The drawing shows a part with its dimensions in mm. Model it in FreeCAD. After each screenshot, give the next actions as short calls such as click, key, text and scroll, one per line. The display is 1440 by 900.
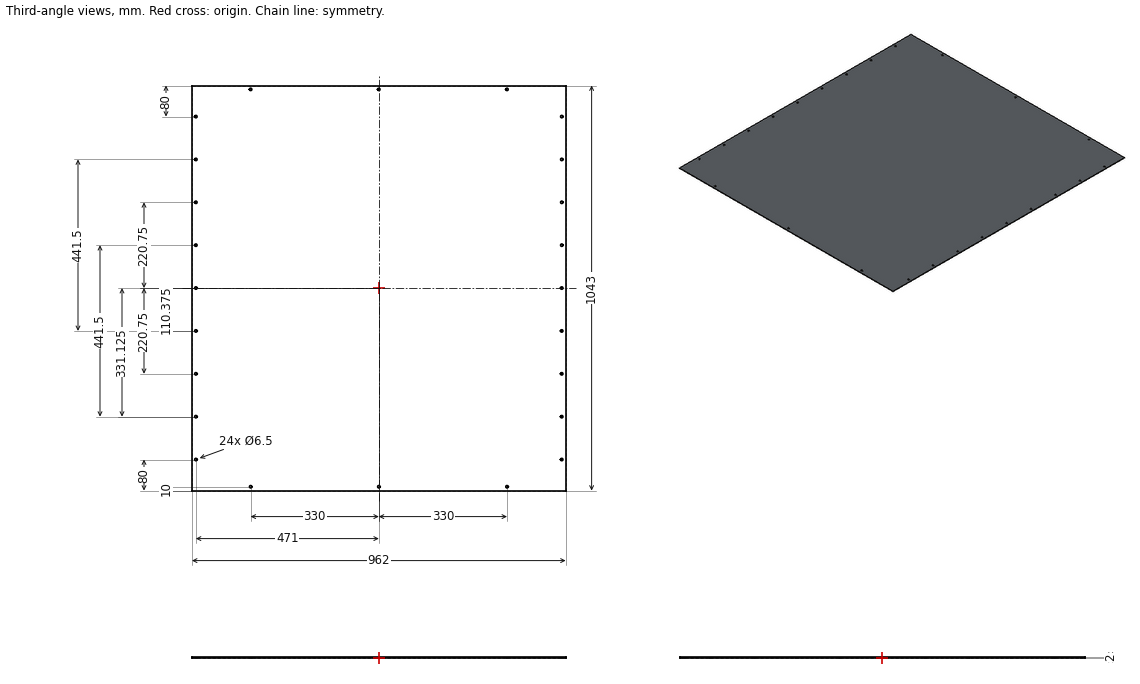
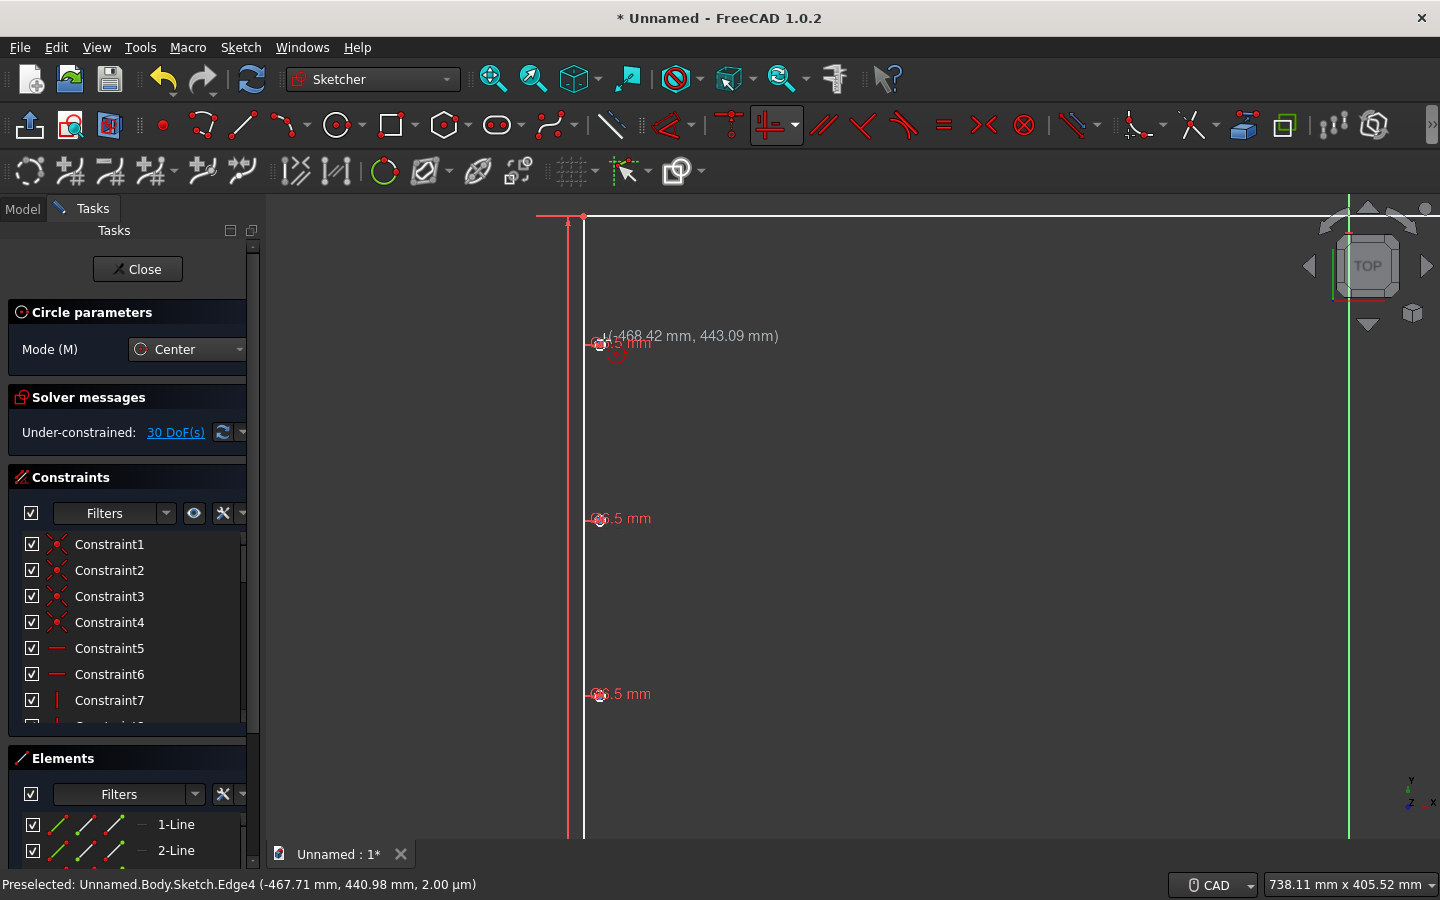
scroll(824, 232, up, 8)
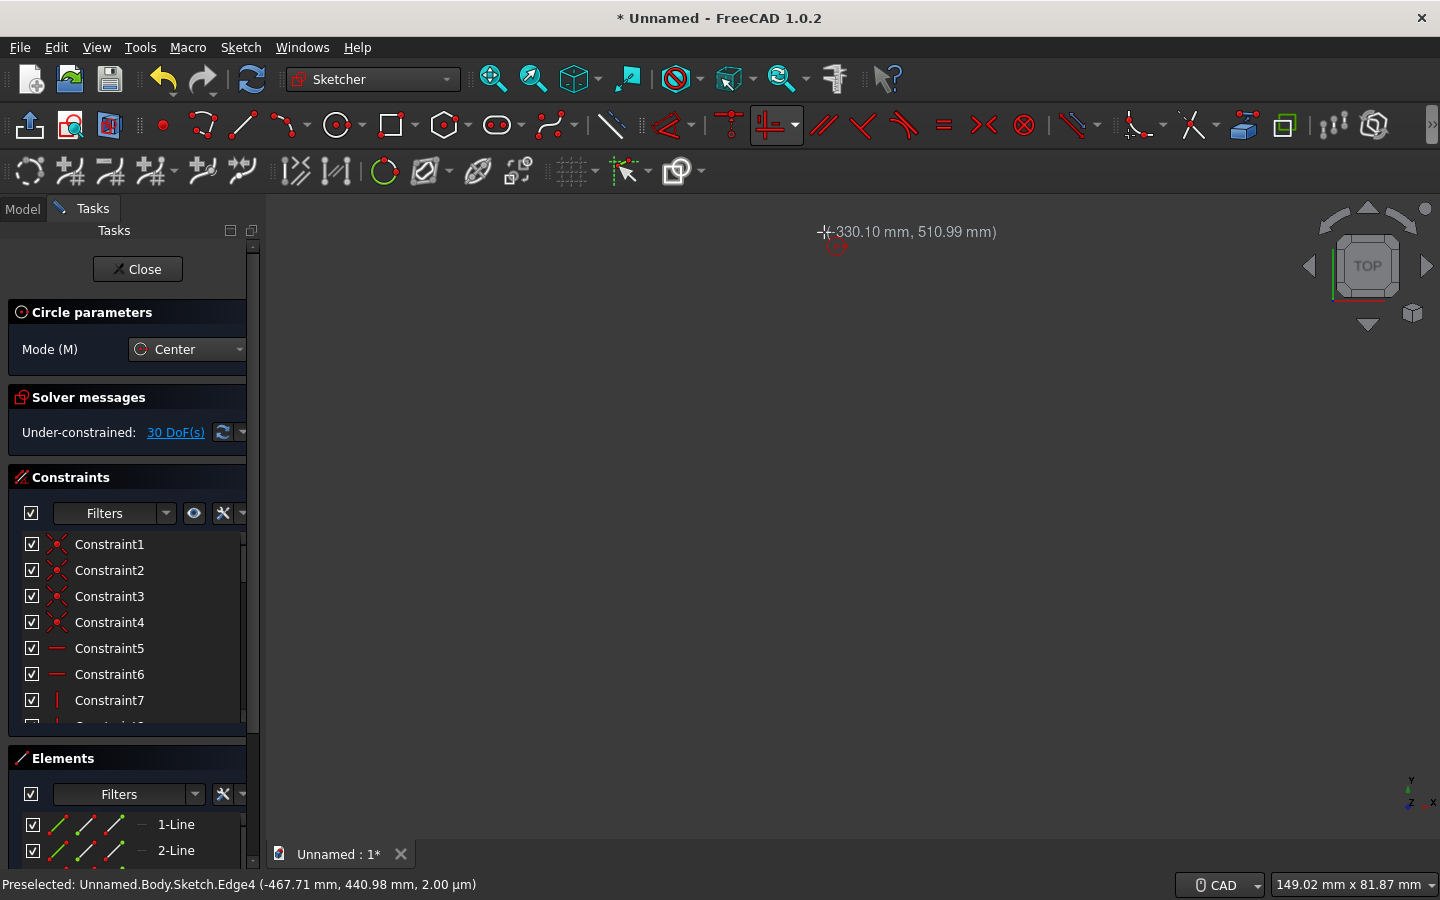
scroll(646, 320, down, 15)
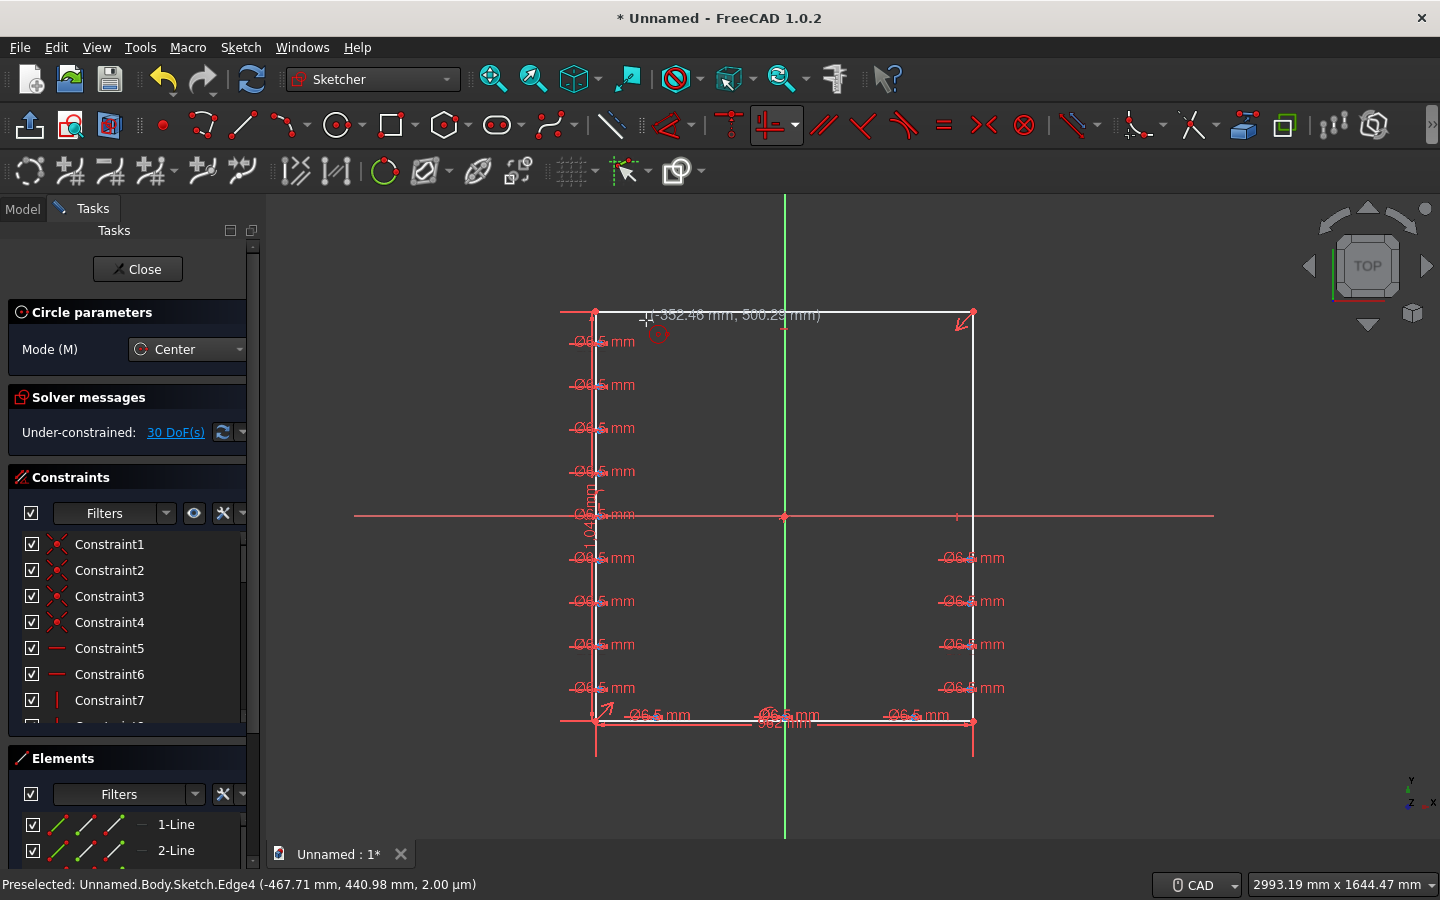
scroll(655, 316, up, 7)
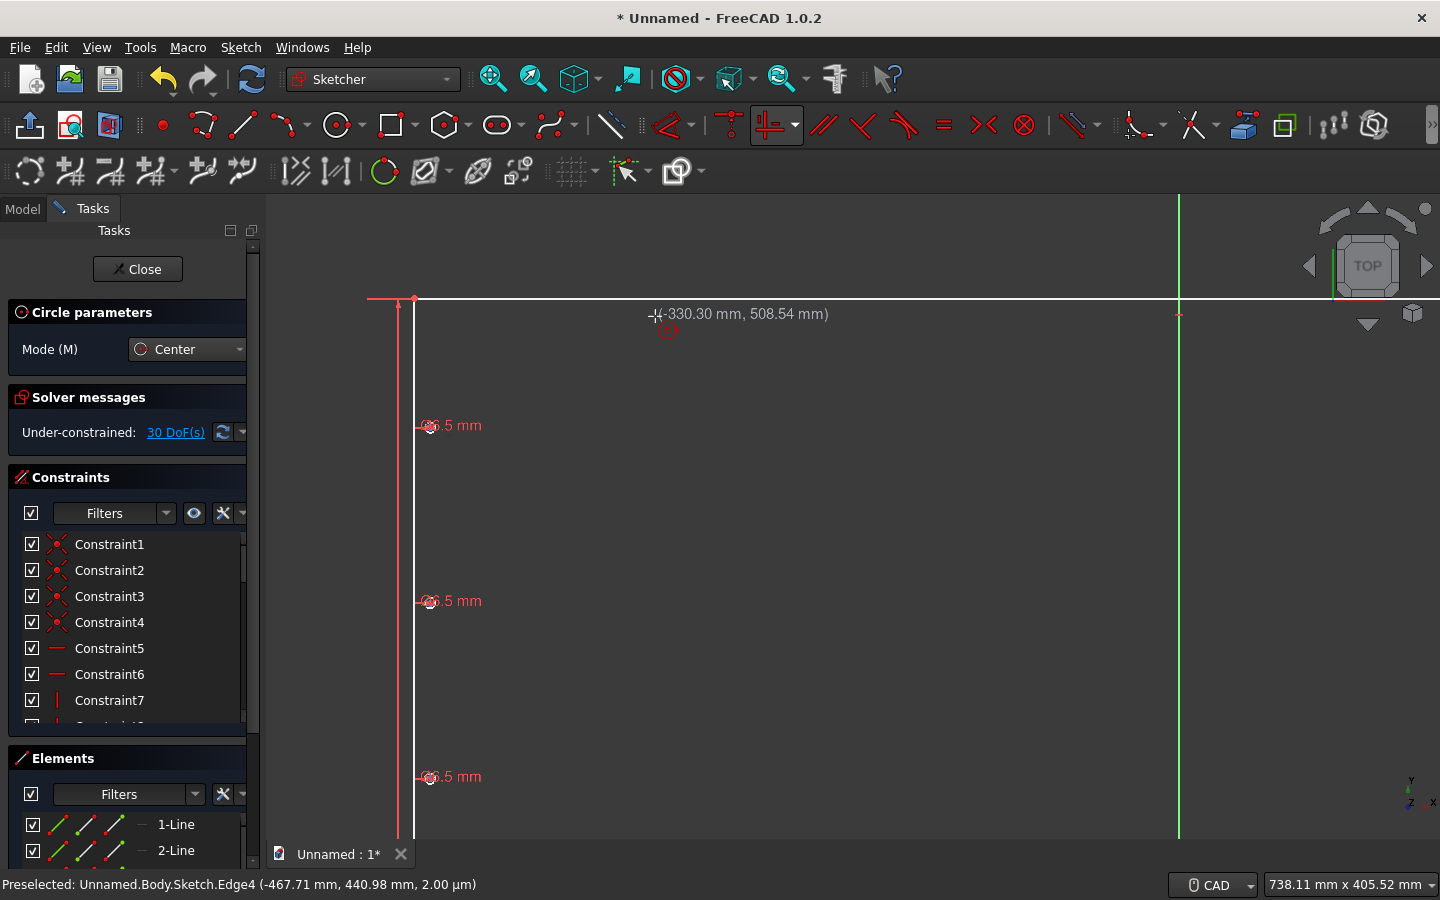
click(654, 315)
move(658, 318)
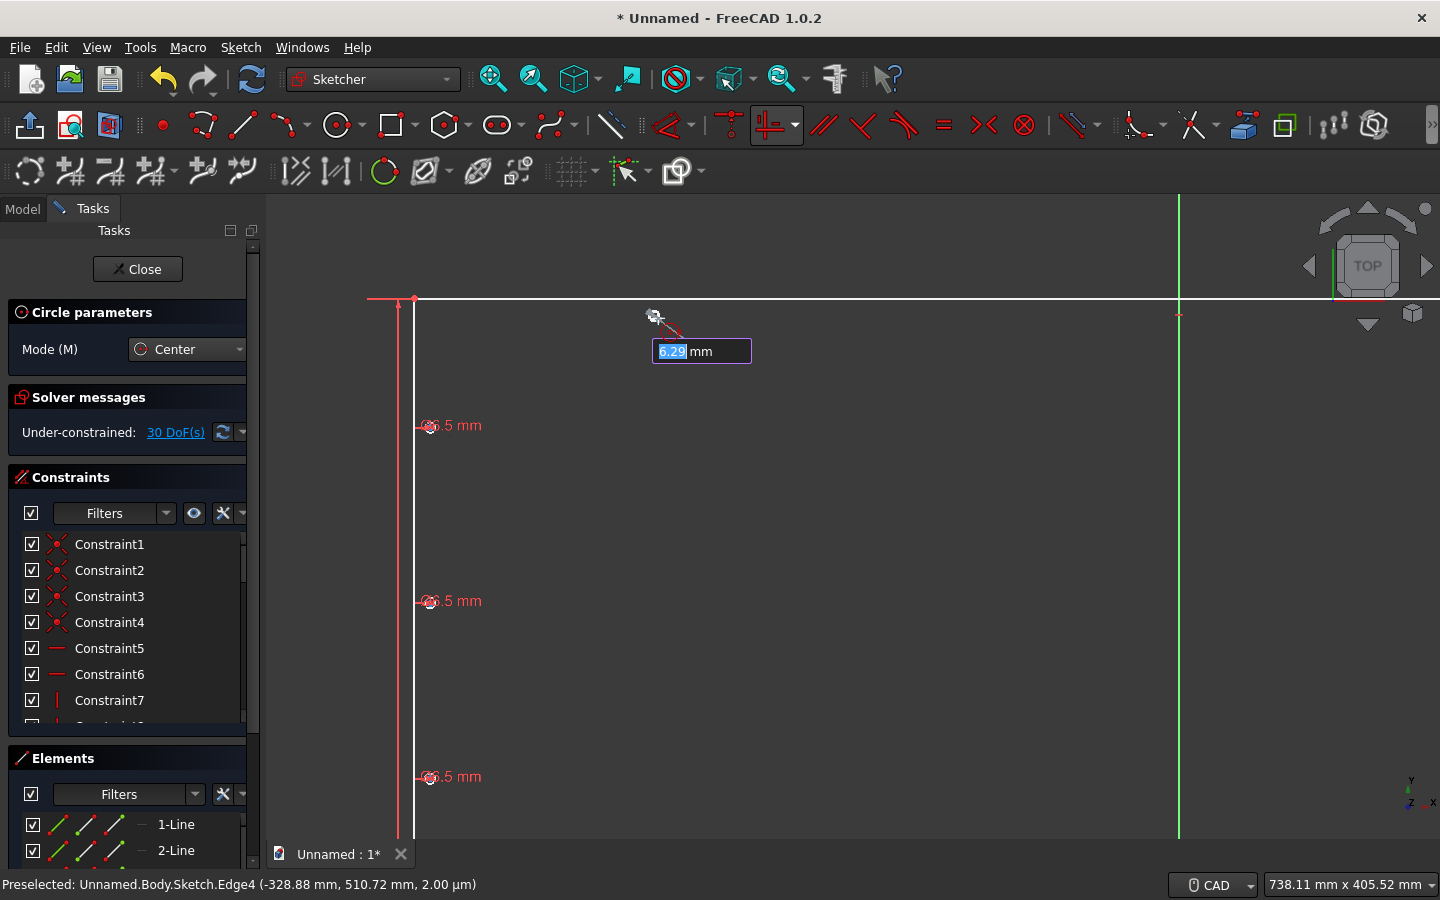
text(6.5)
key(Return)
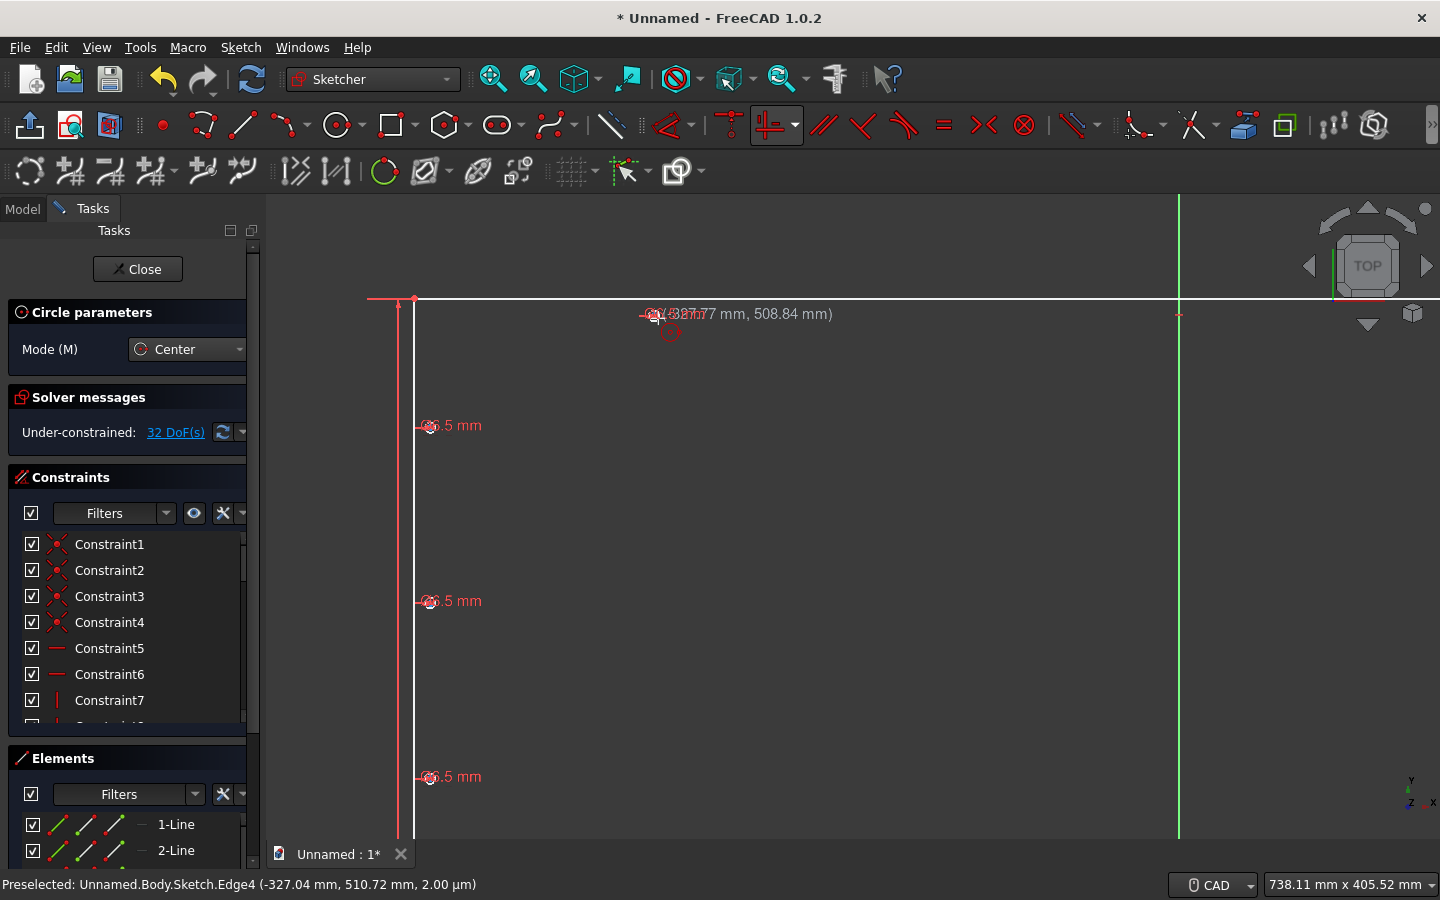
scroll(655, 316, down, 7)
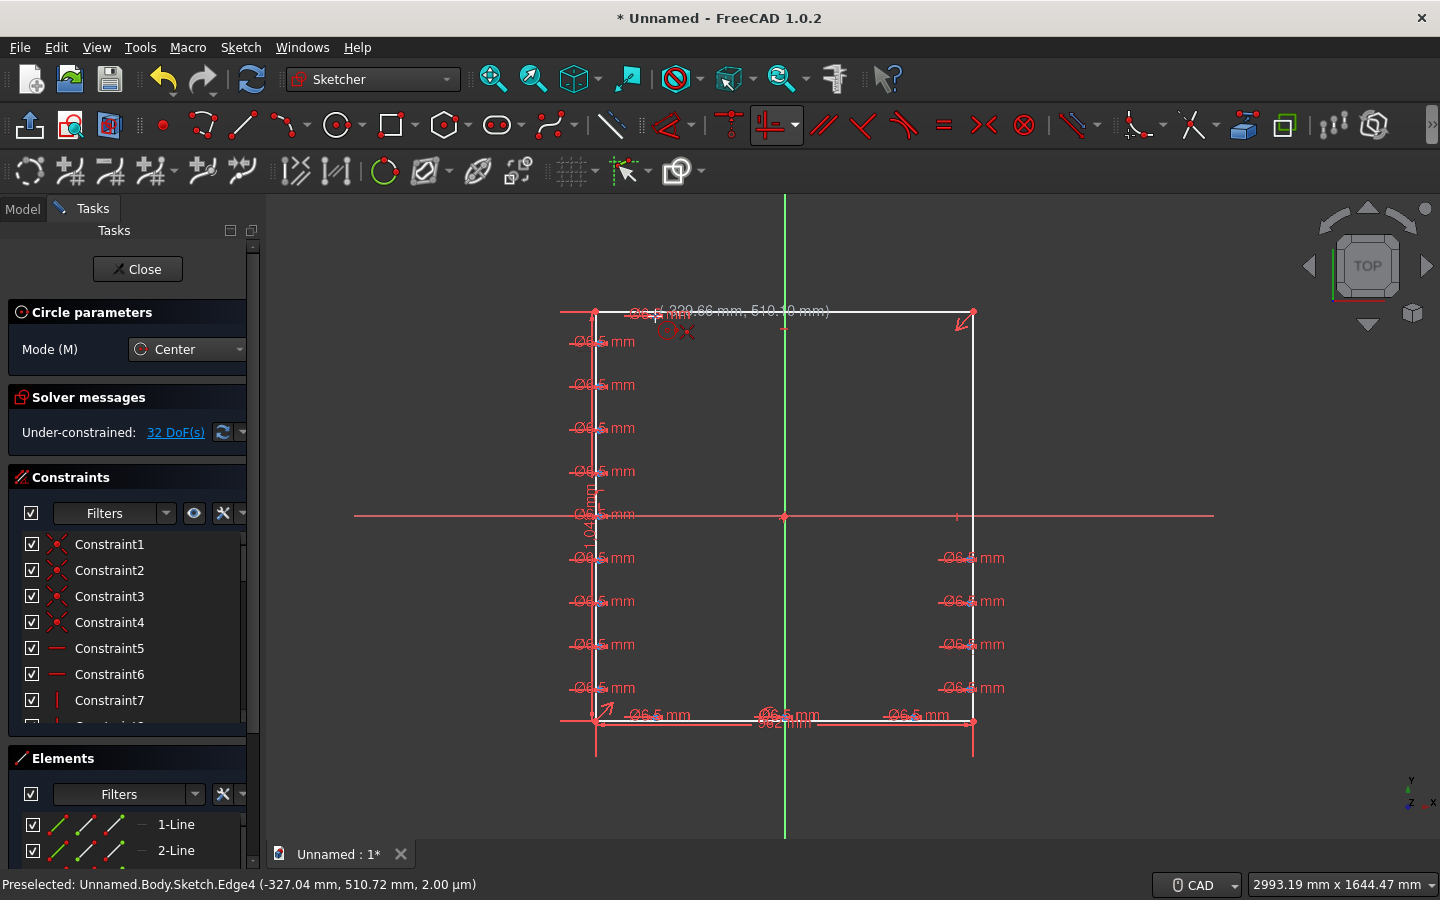
scroll(969, 516, up, 15)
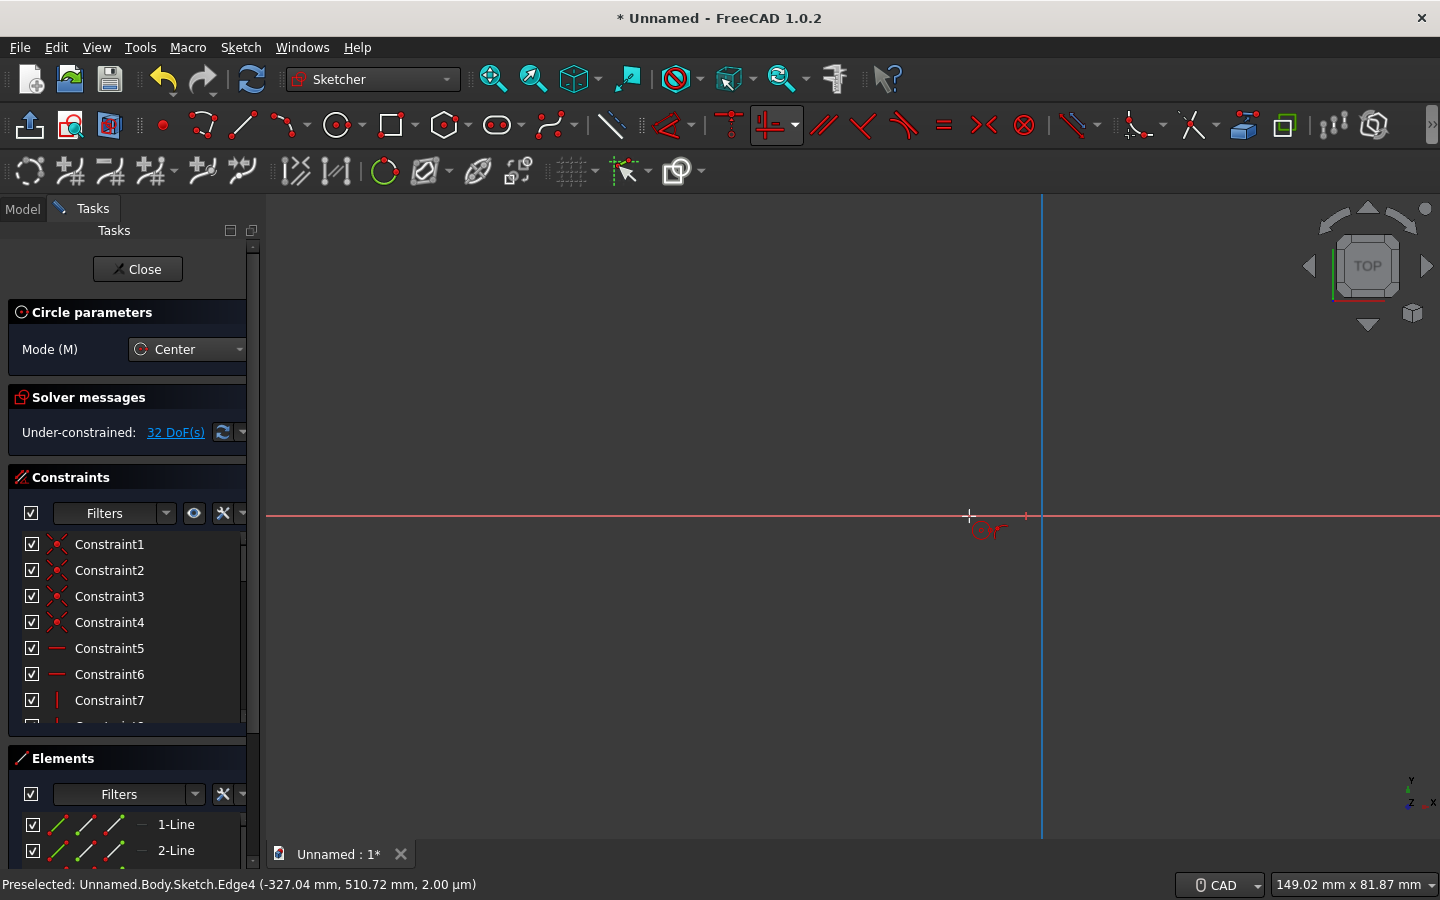
scroll(970, 517, down, 15)